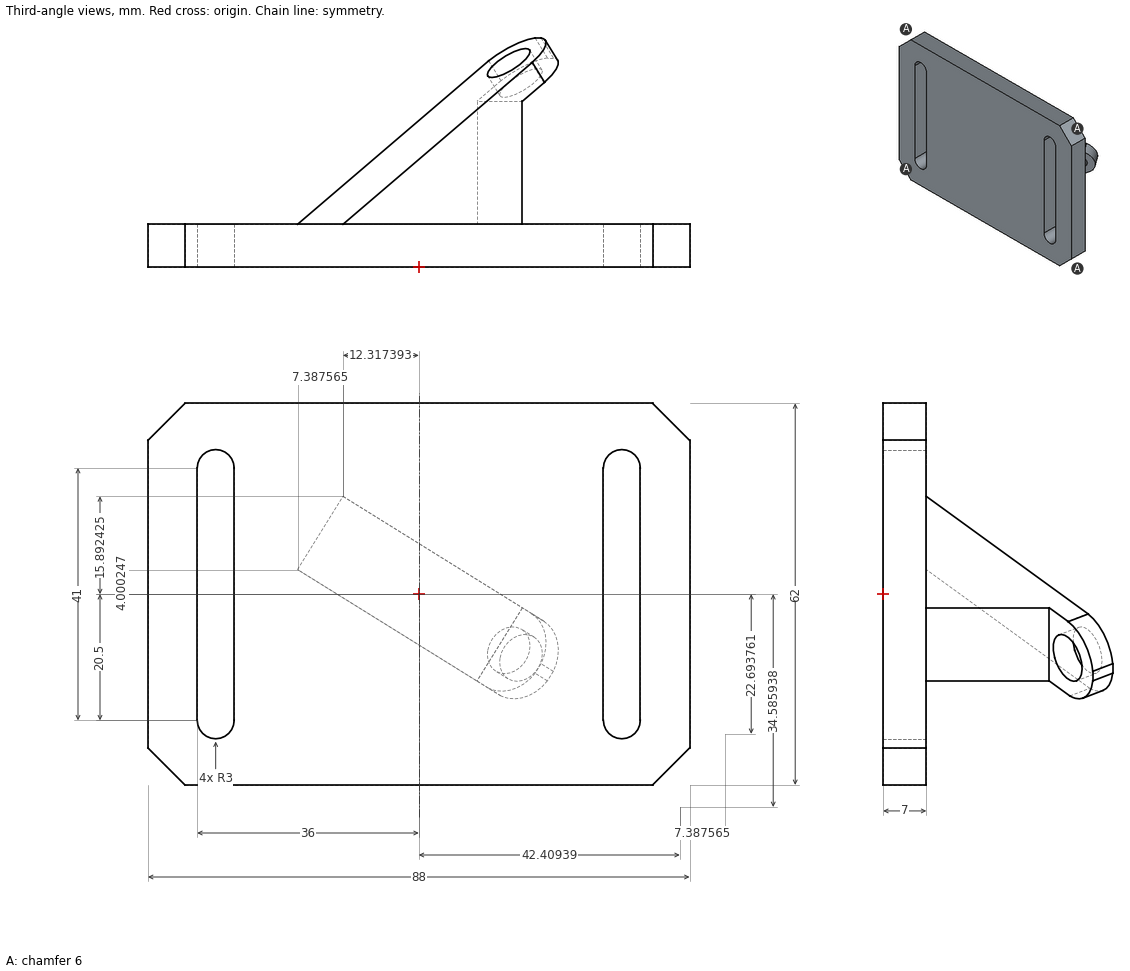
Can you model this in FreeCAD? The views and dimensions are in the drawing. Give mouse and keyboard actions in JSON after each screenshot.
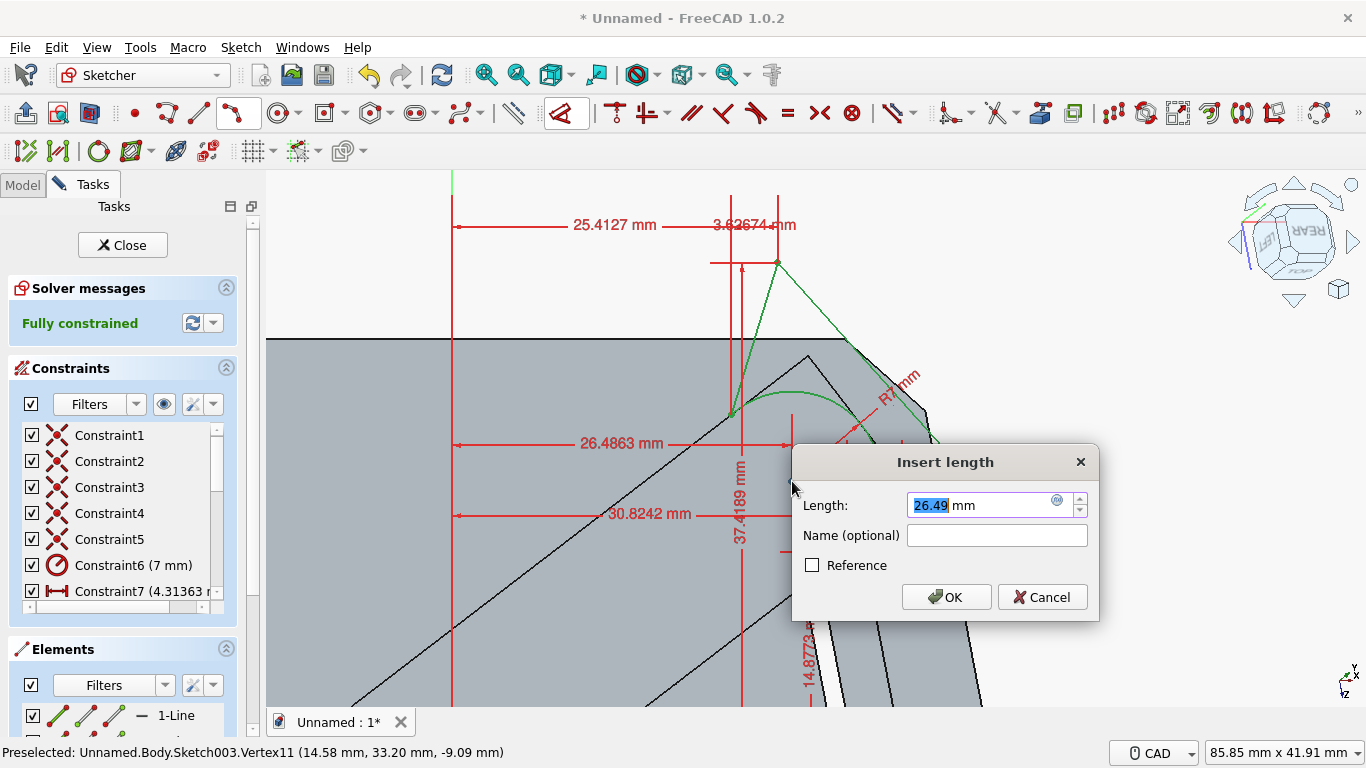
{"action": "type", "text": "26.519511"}
{"action": "key", "text": "Return"}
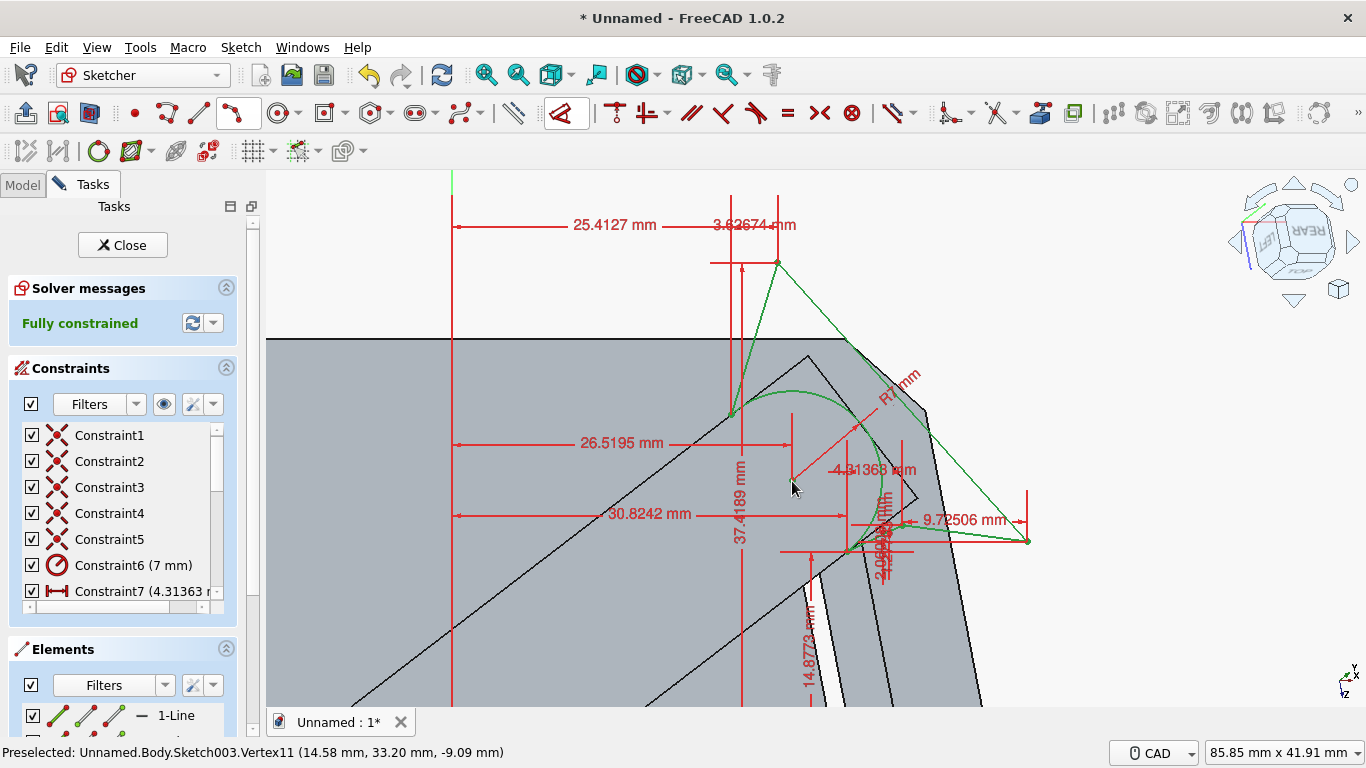
{"action": "left_click", "coordinate": [123, 245]}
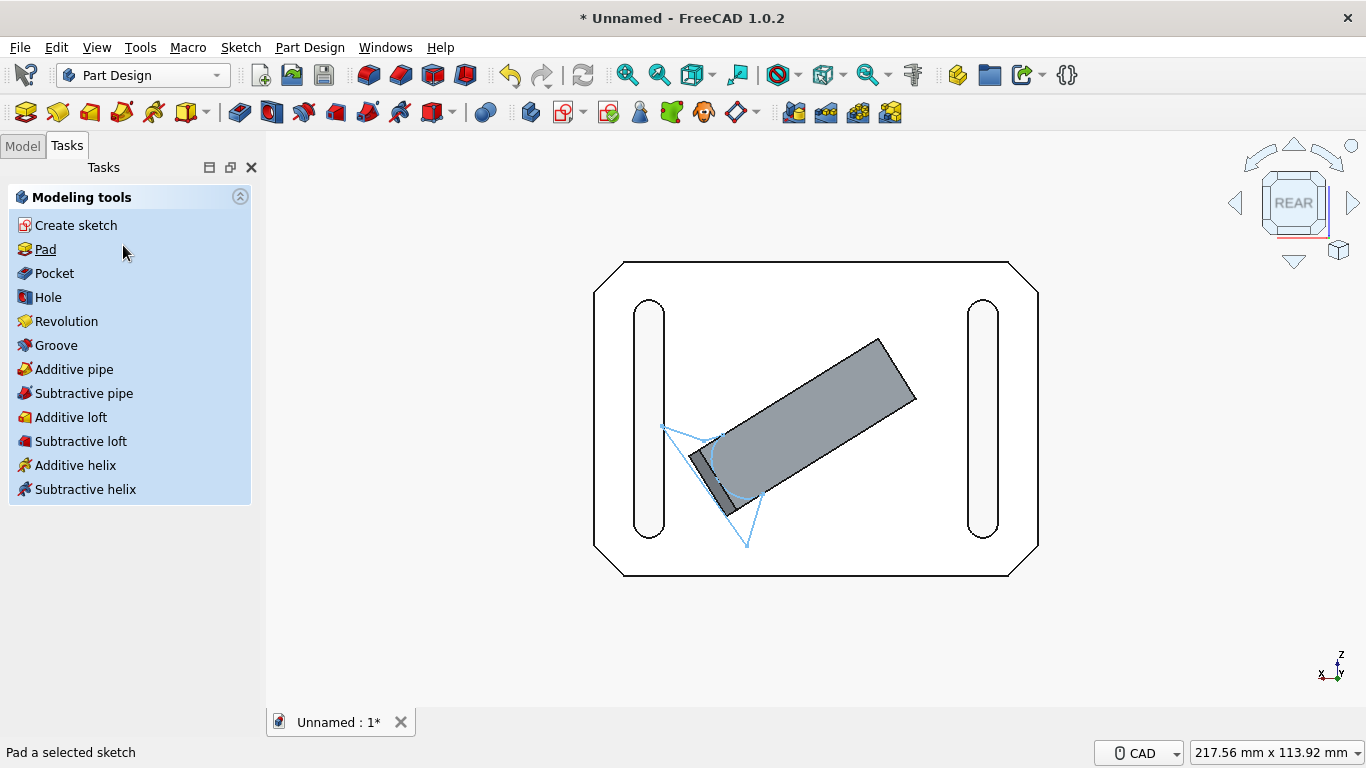
{"action": "left_click", "coordinate": [240, 112]}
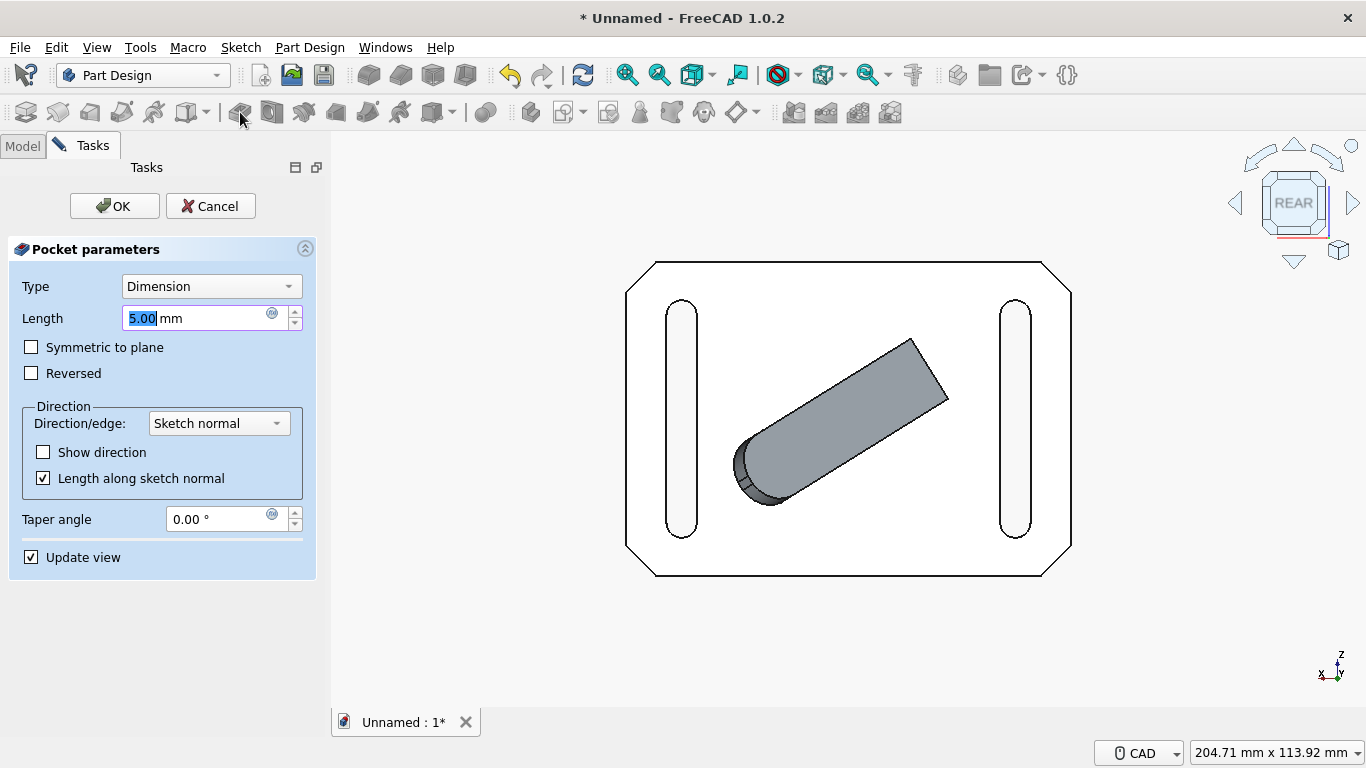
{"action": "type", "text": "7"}
{"action": "key", "text": "Tab"}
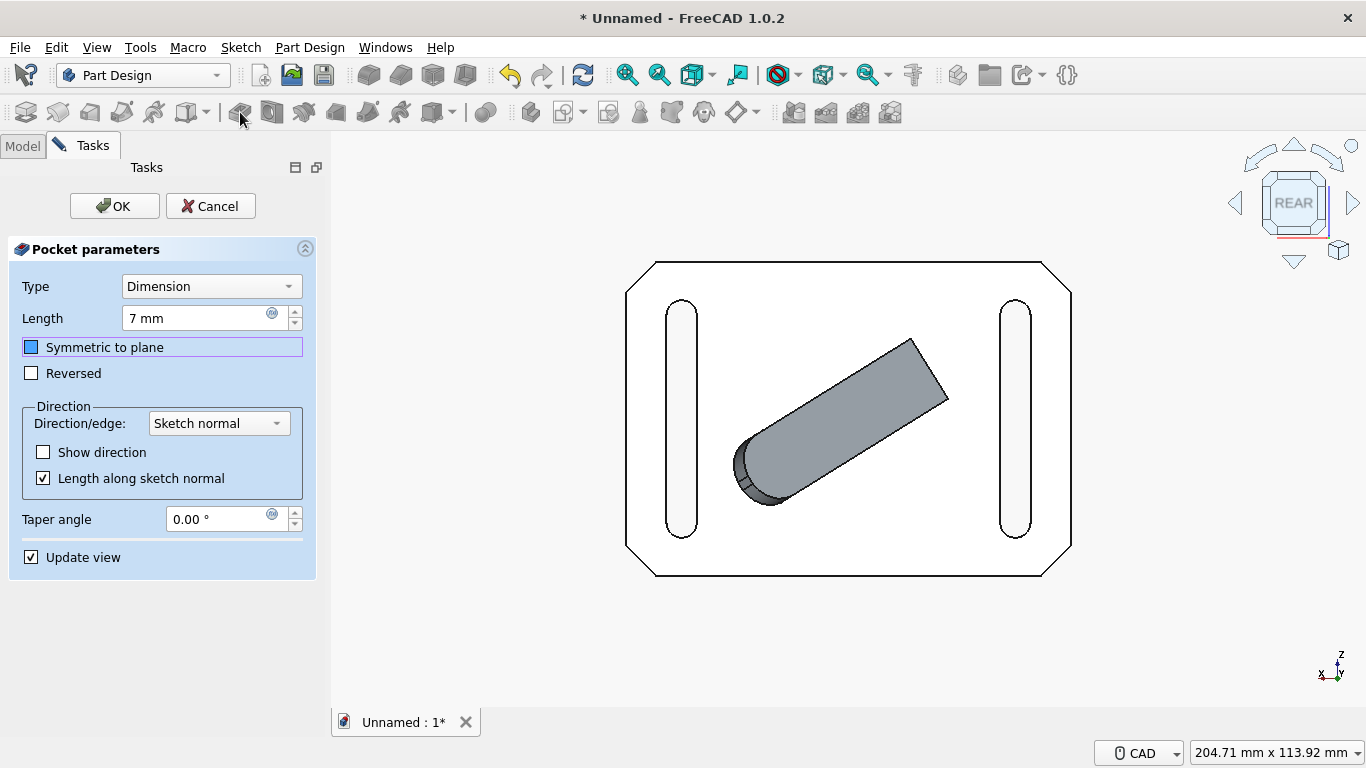
{"action": "left_click", "coordinate": [115, 206]}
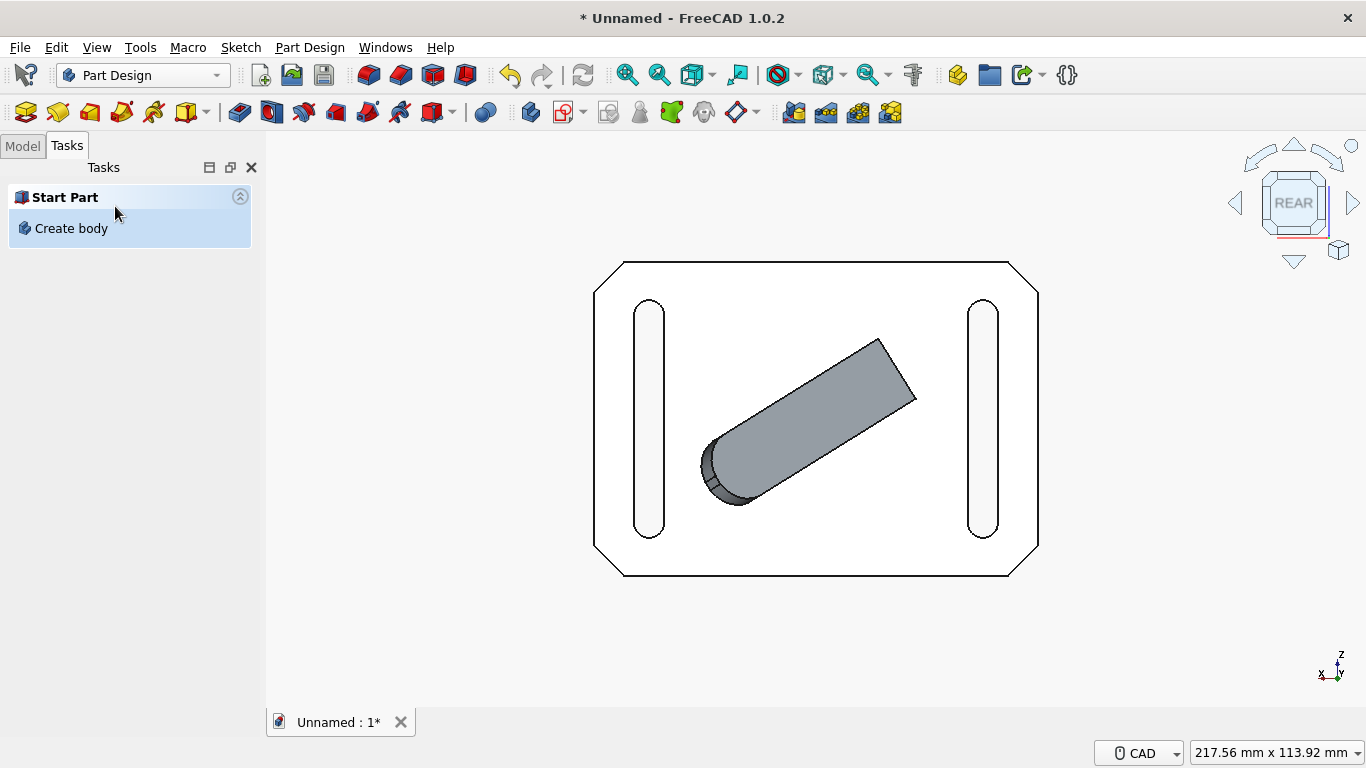
{"action": "left_click", "coordinate": [859, 392]}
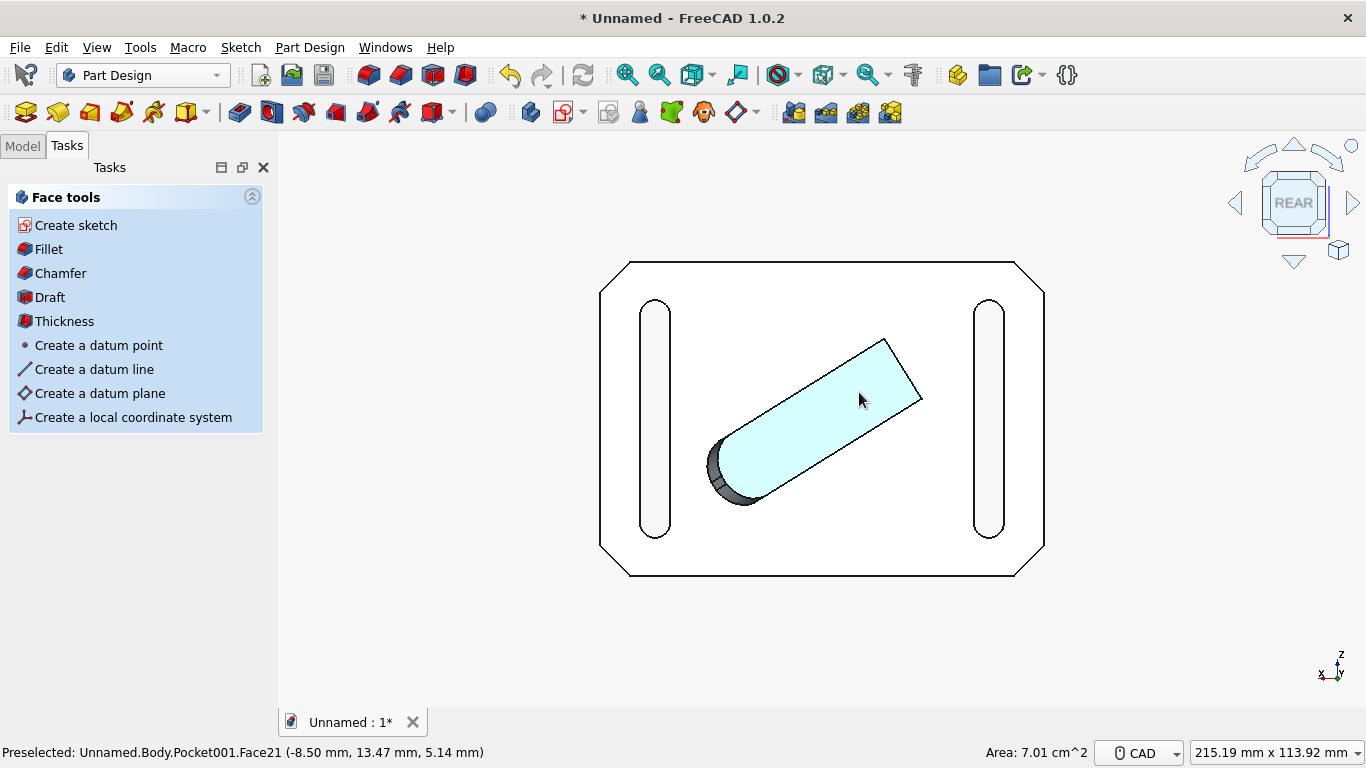
{"action": "left_click", "coordinate": [564, 112]}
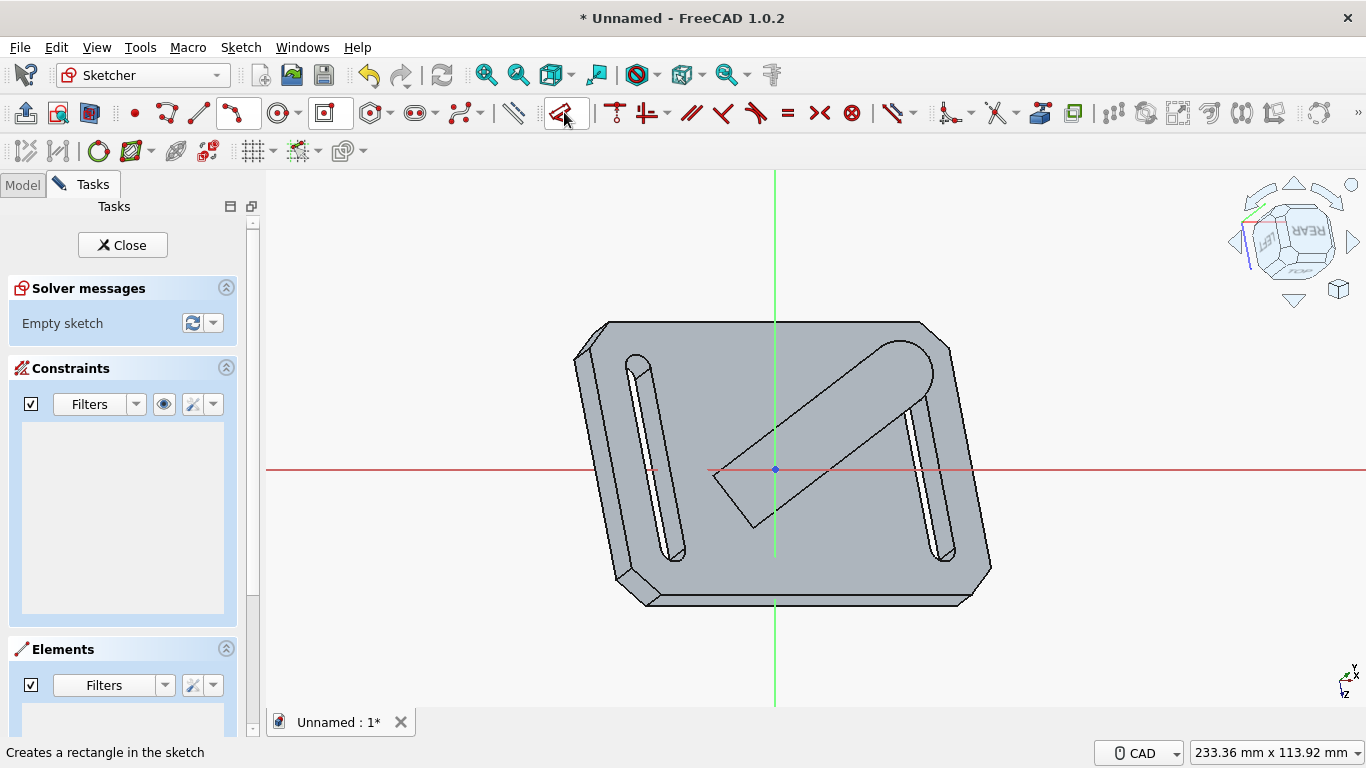
{"action": "scroll", "coordinate": [919, 366], "scroll_direction": "up", "scroll_amount": 11}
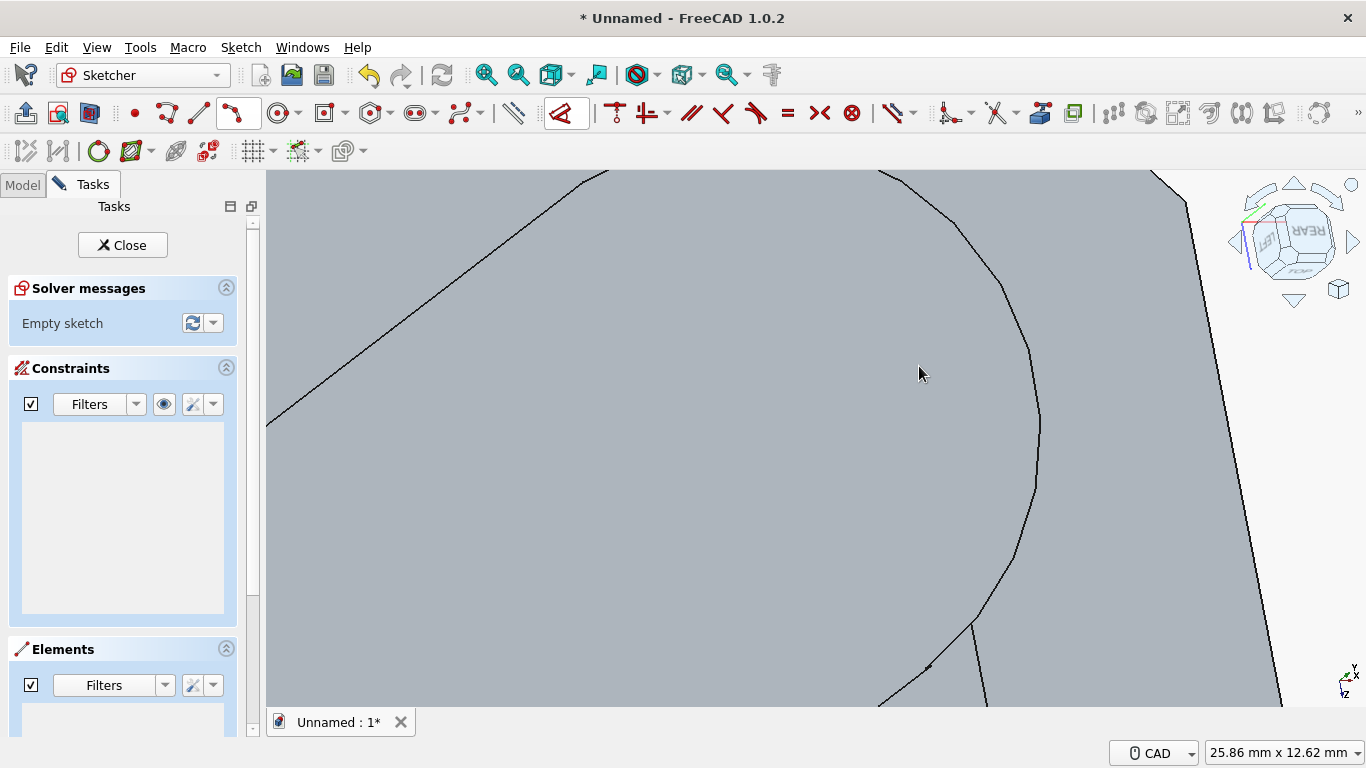
{"action": "left_click", "coordinate": [278, 114]}